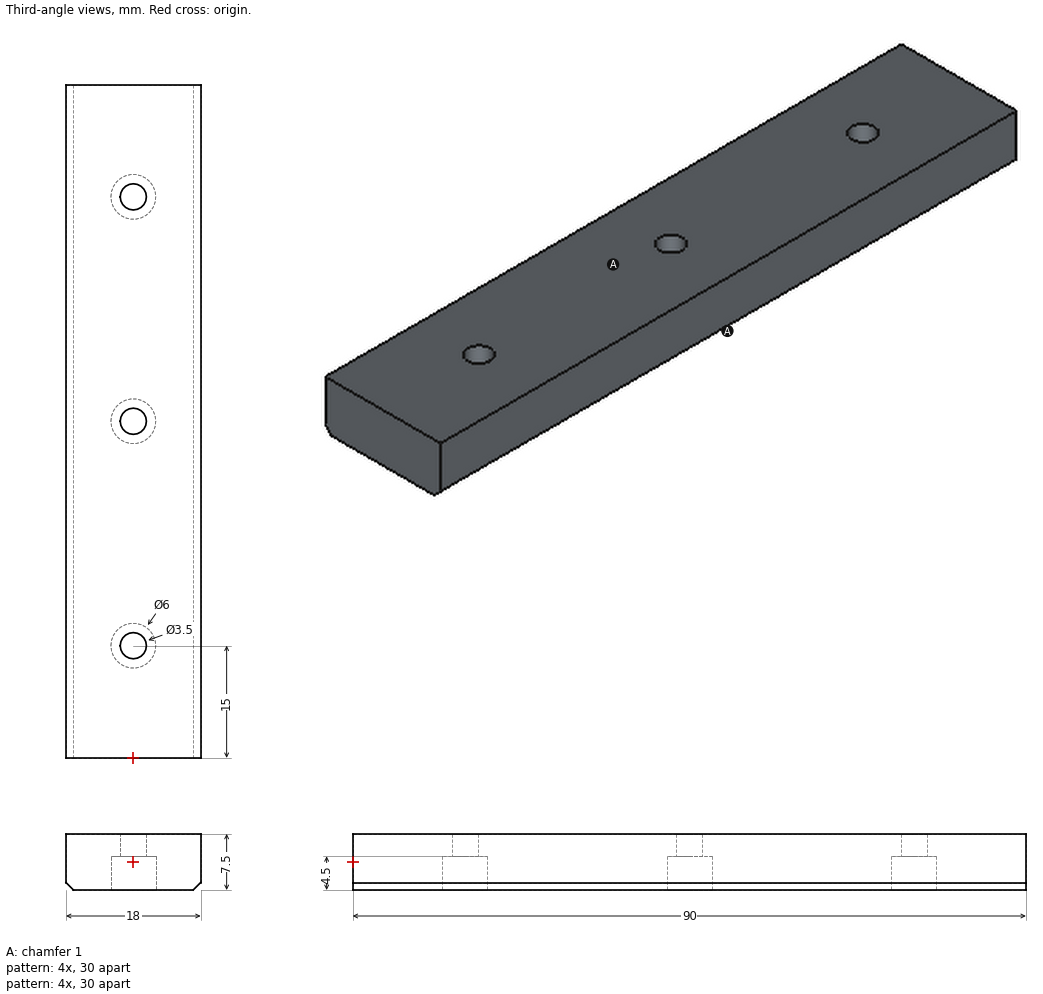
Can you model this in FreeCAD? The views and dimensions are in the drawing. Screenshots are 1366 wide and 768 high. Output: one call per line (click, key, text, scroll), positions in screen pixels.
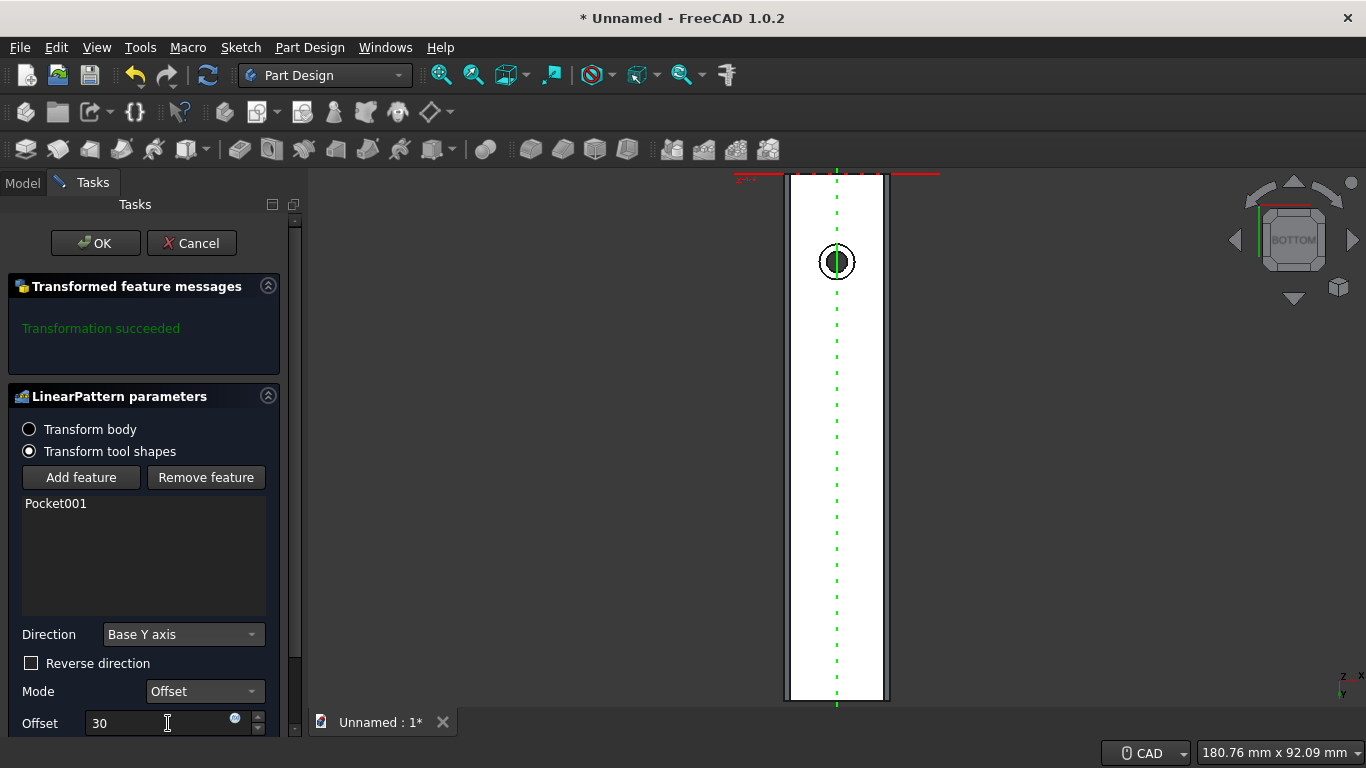
scroll(295, 475, down, 2)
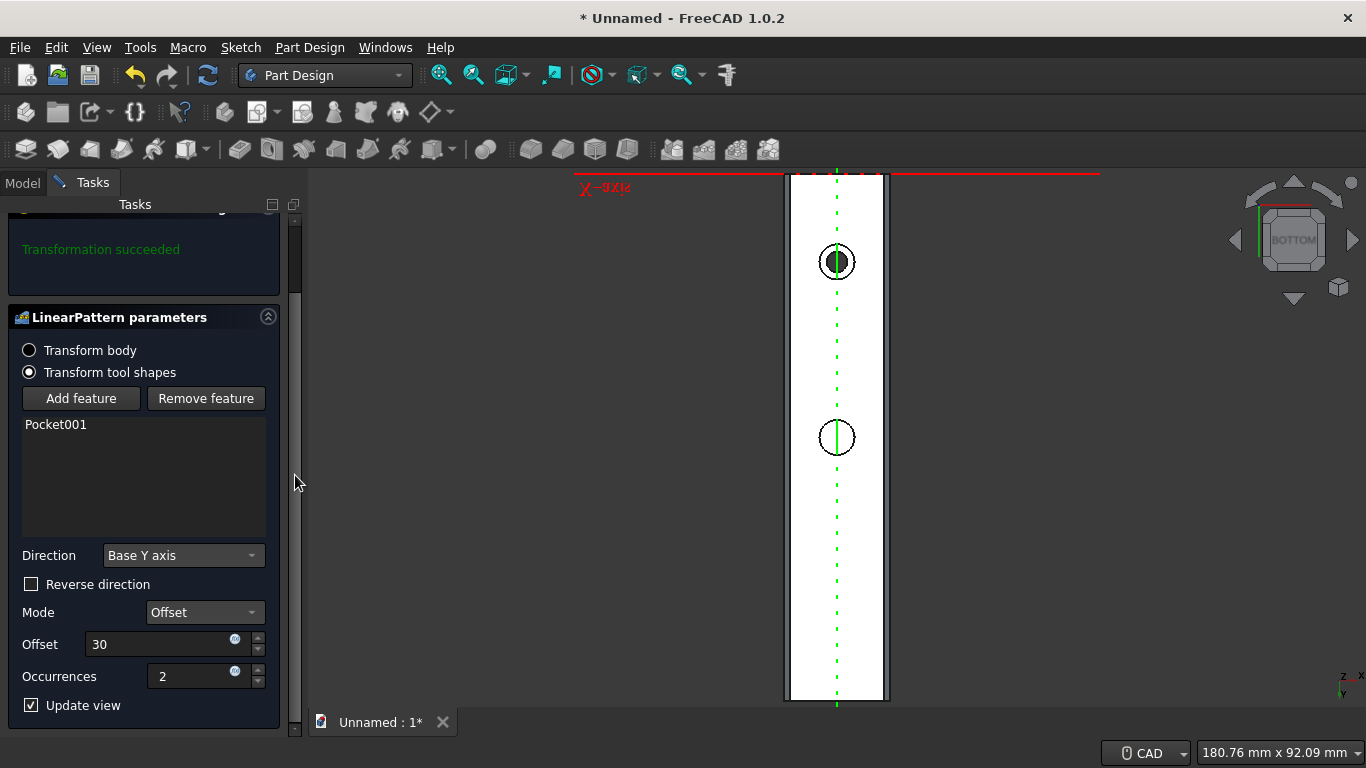
triple_click(198, 676)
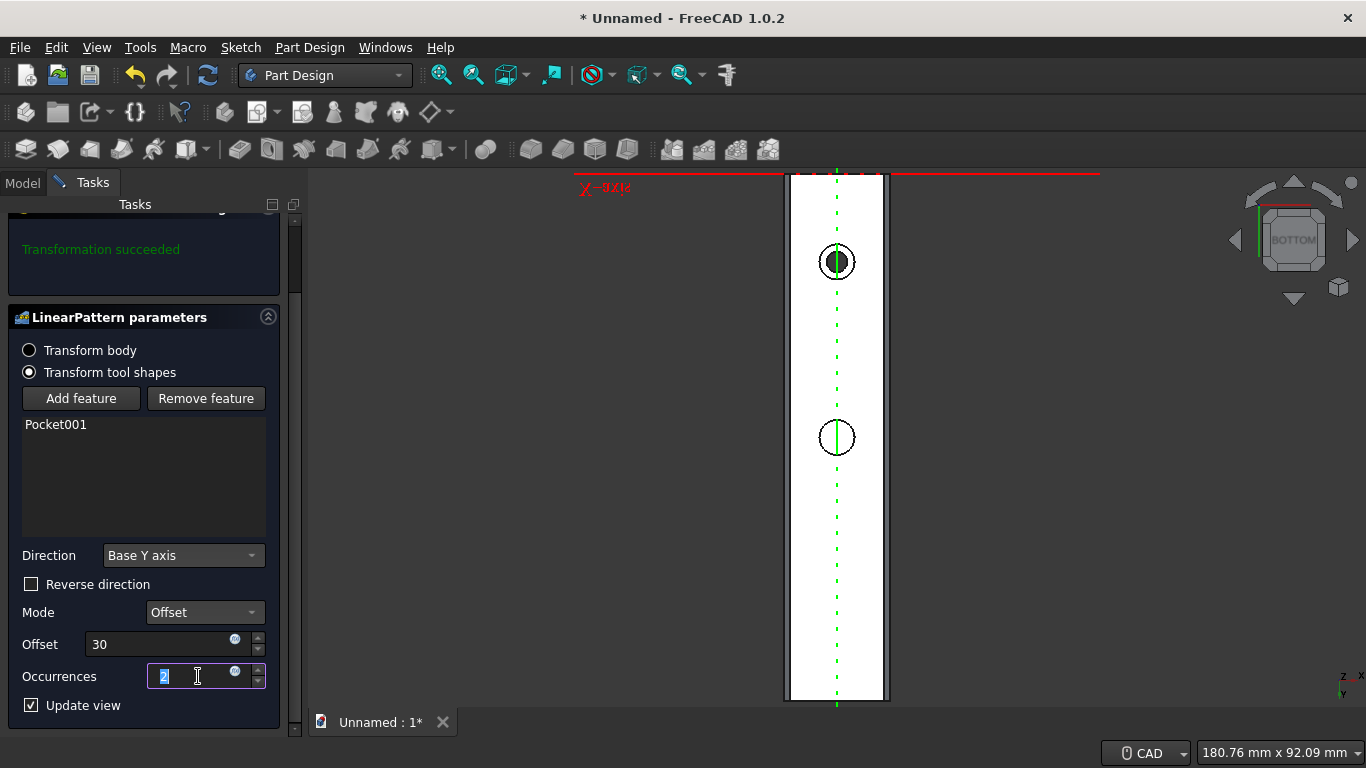
text(4)
key(Tab)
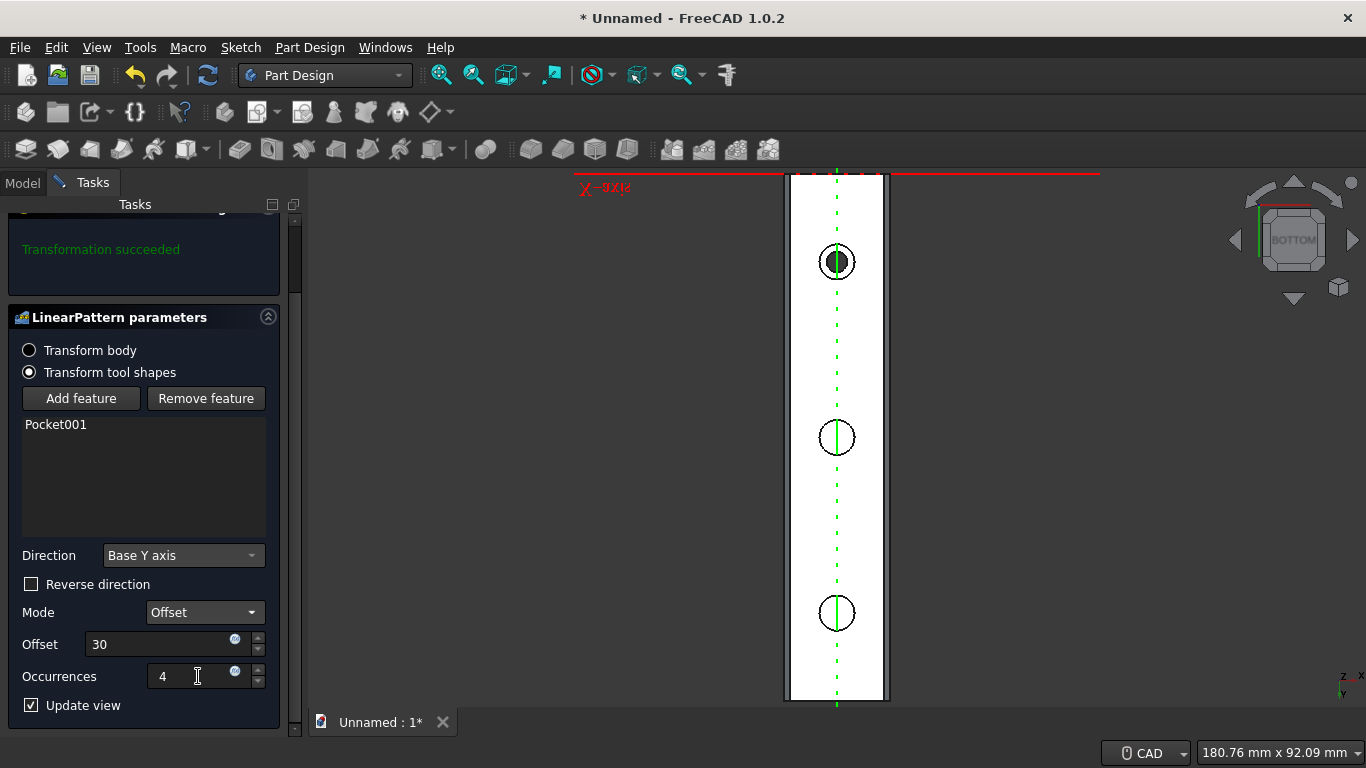
scroll(295, 475, up, 3)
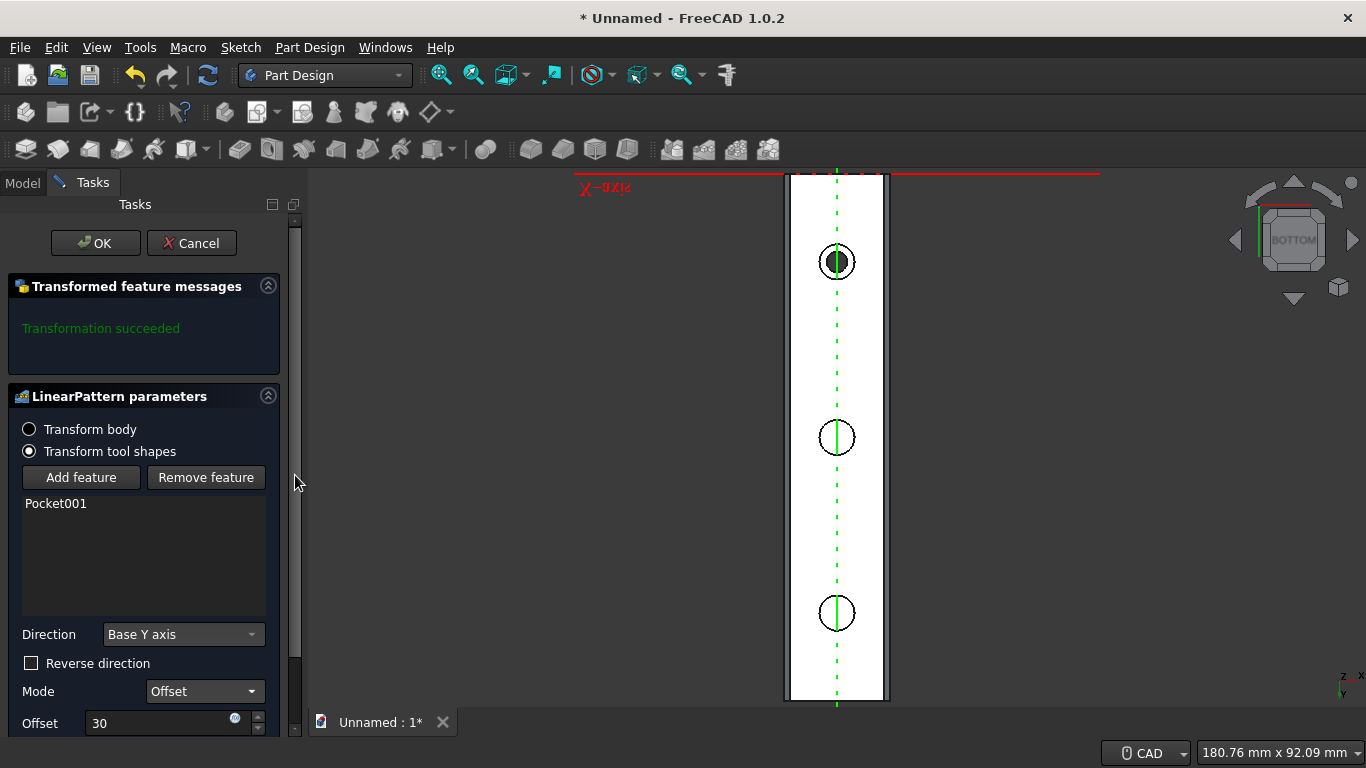
click(96, 243)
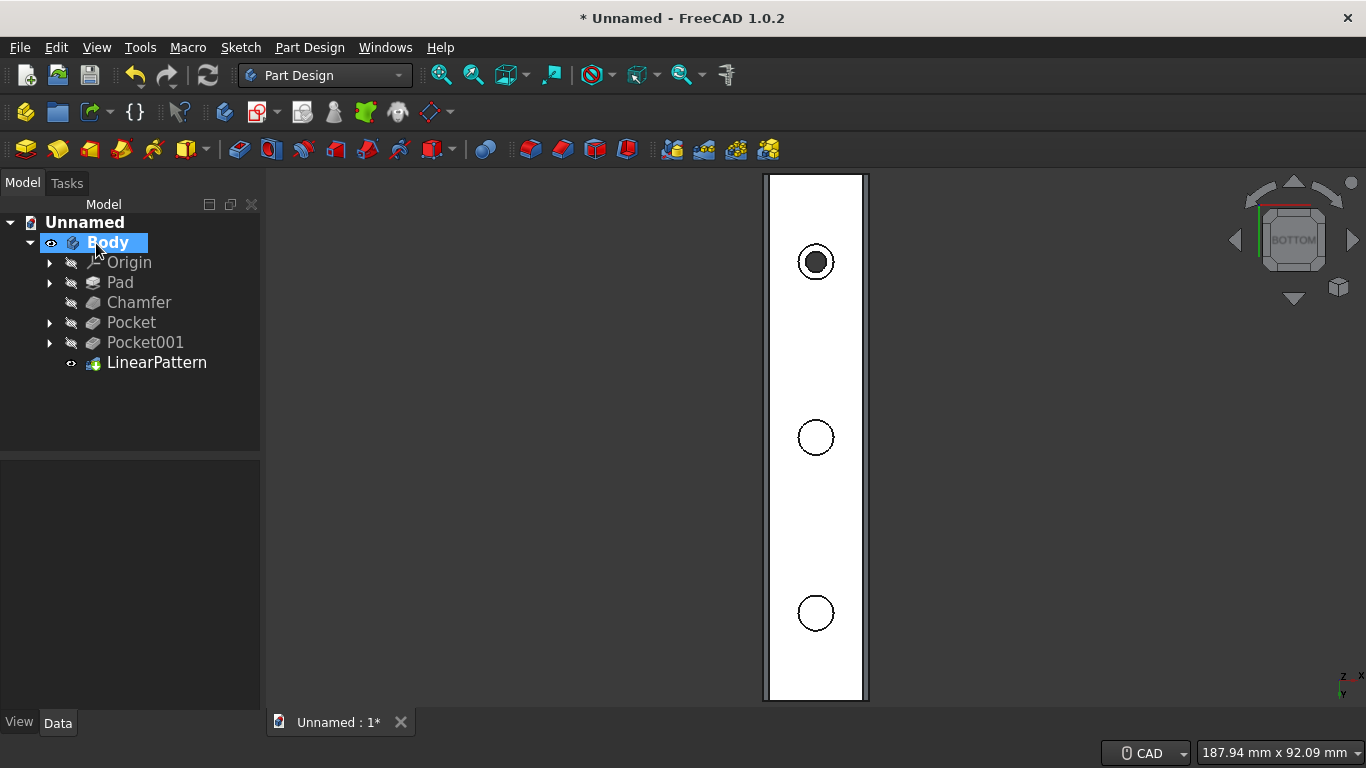
click(116, 323)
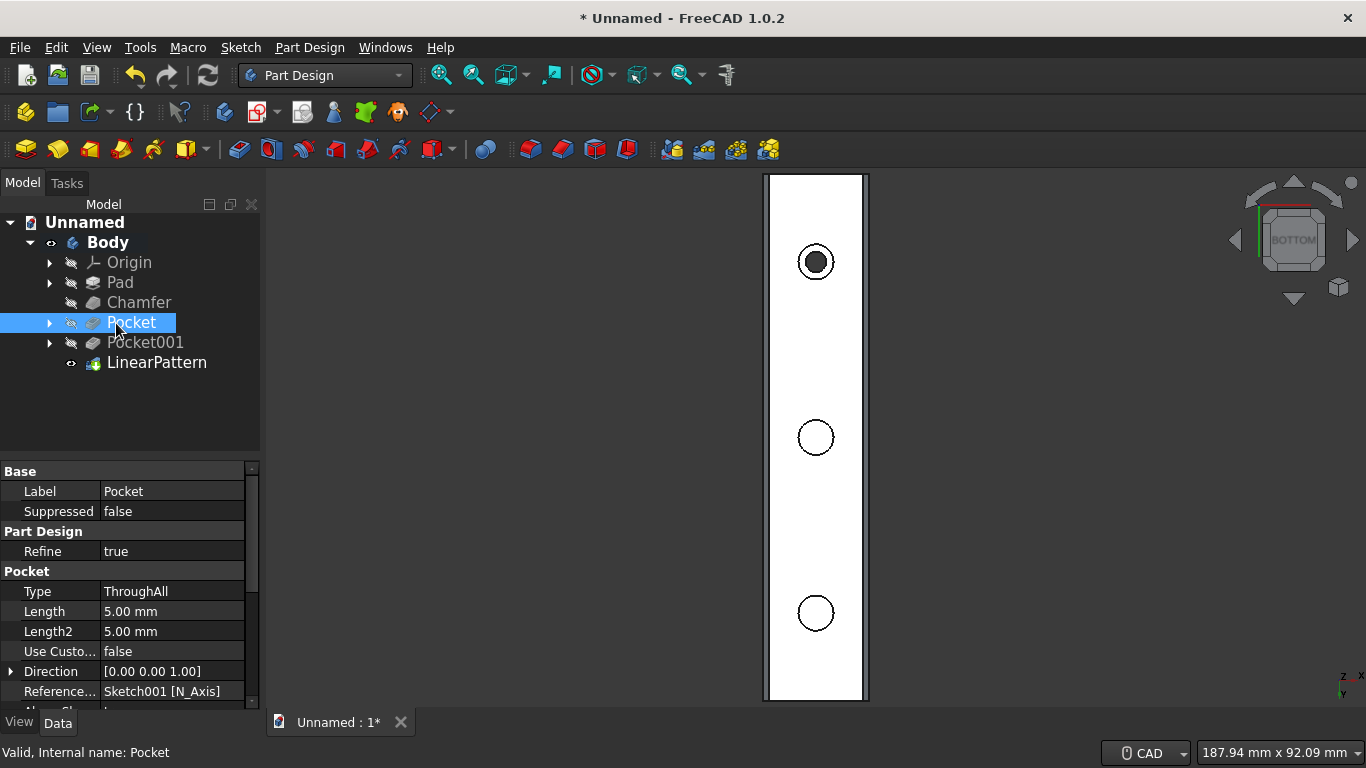
click(704, 150)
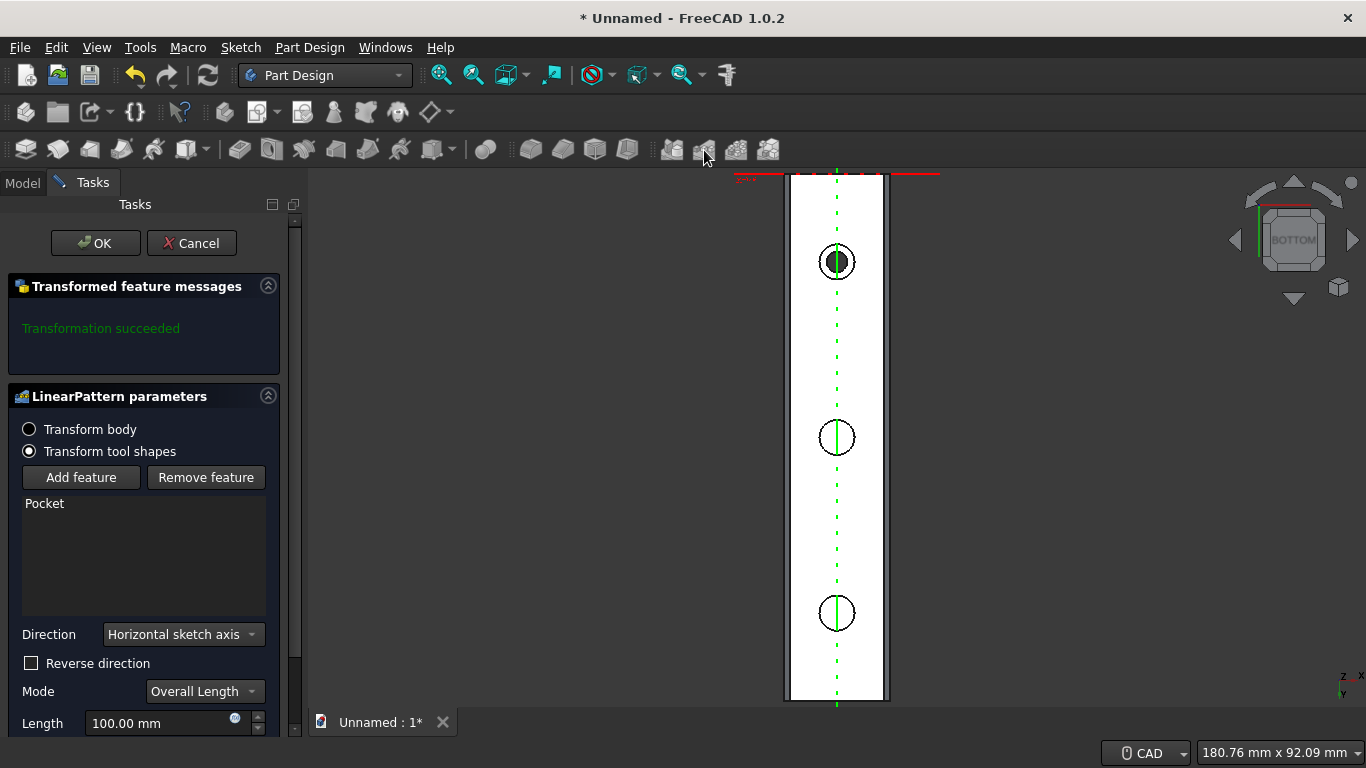
click(184, 634)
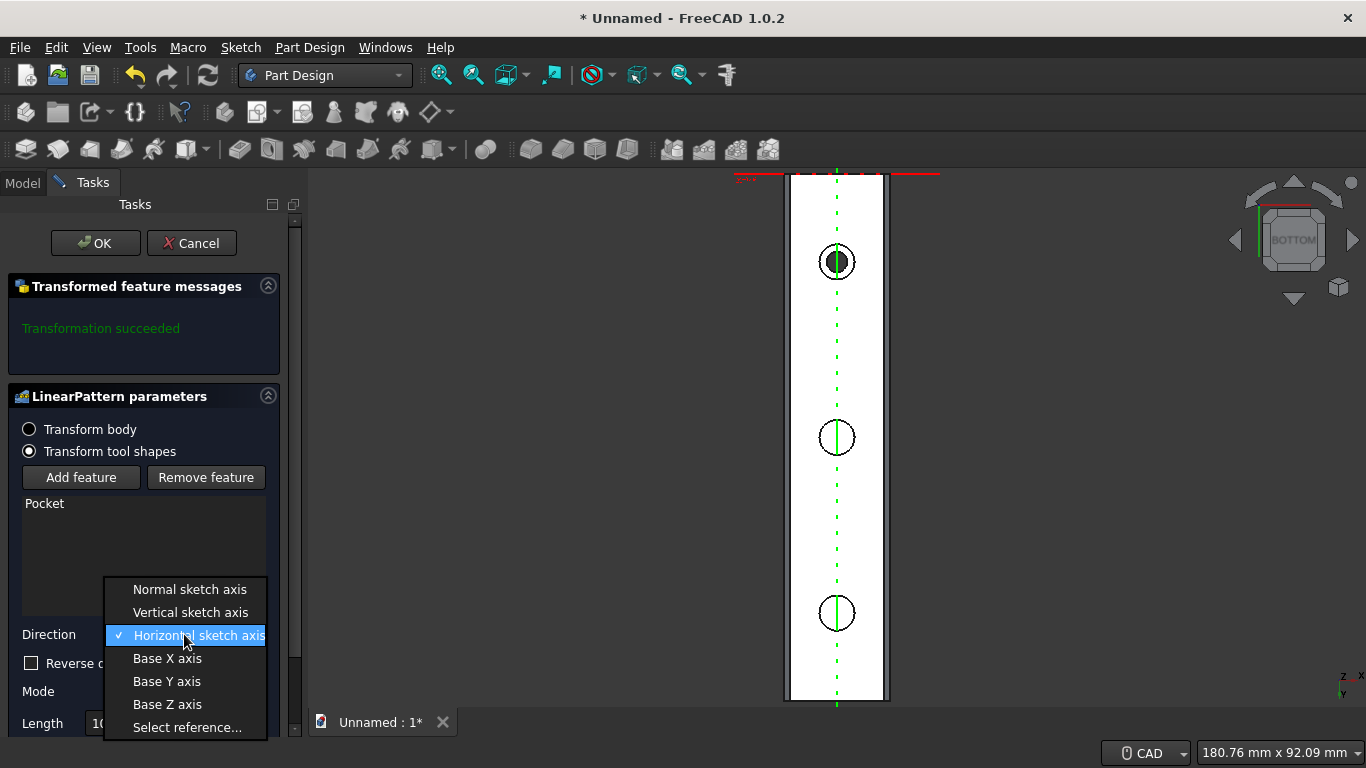
click(184, 682)